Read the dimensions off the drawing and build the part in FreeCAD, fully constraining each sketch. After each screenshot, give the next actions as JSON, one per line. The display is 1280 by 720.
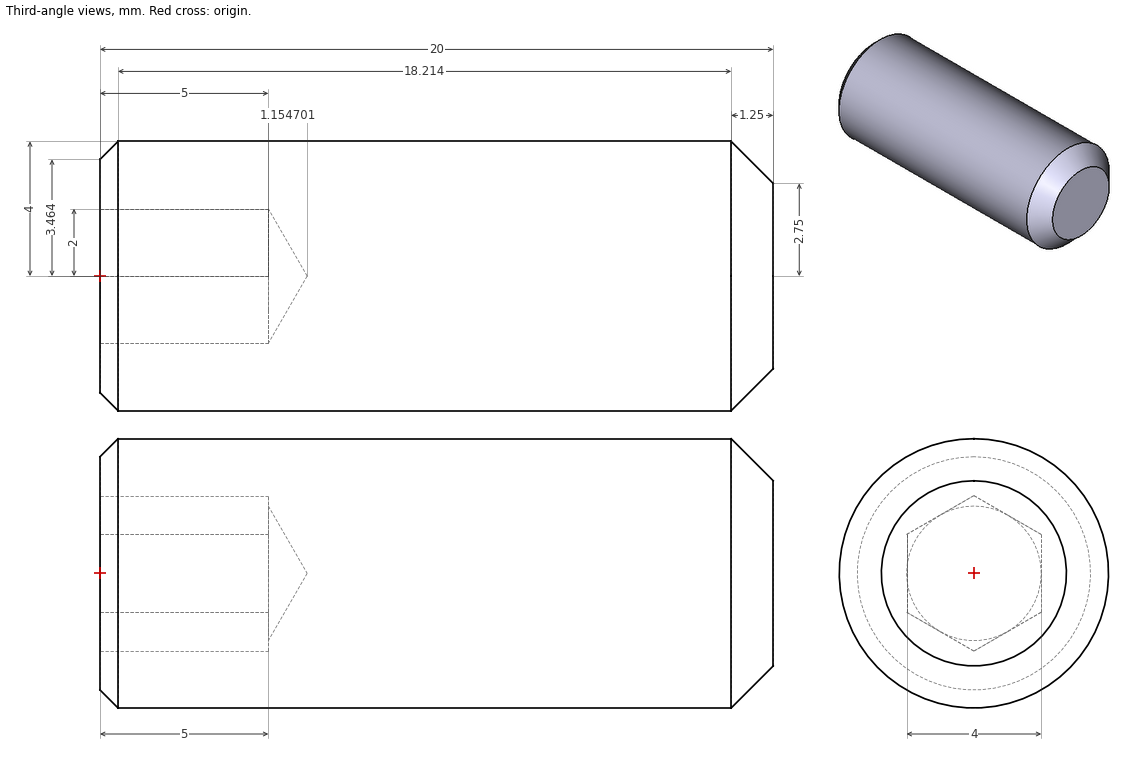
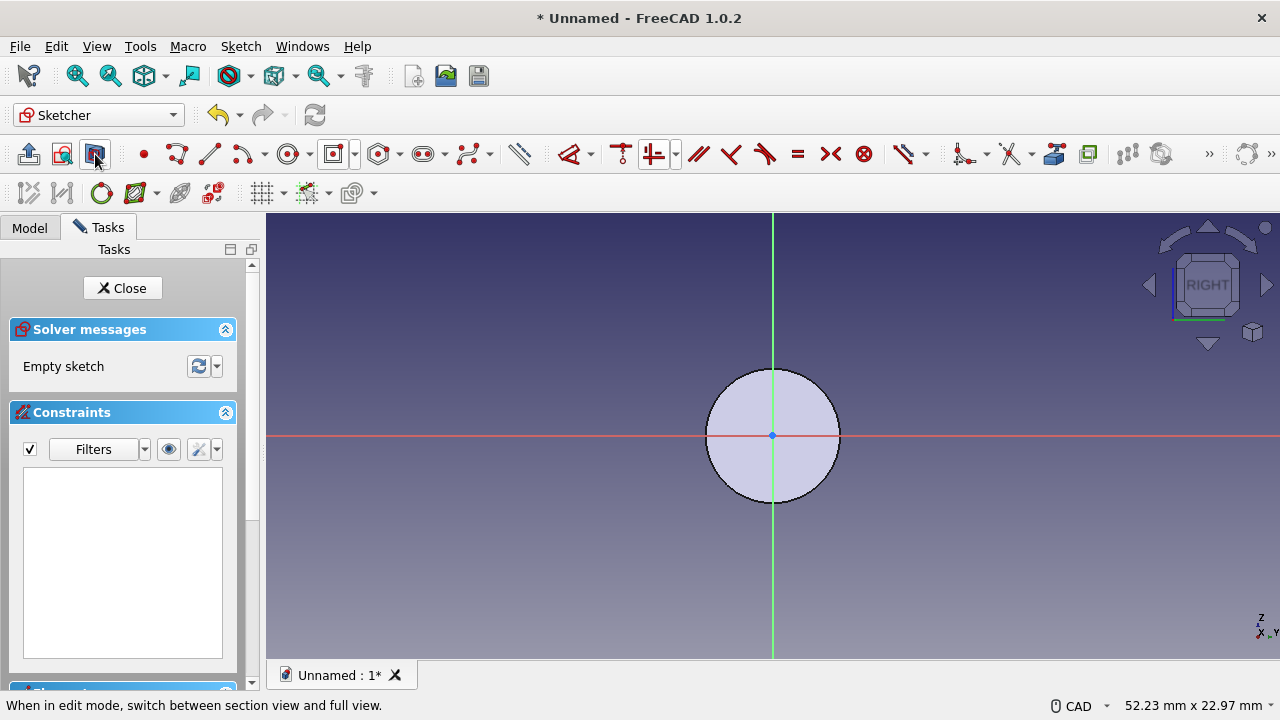
{"action": "scroll", "coordinate": [802, 436], "scroll_direction": "up", "scroll_amount": 6}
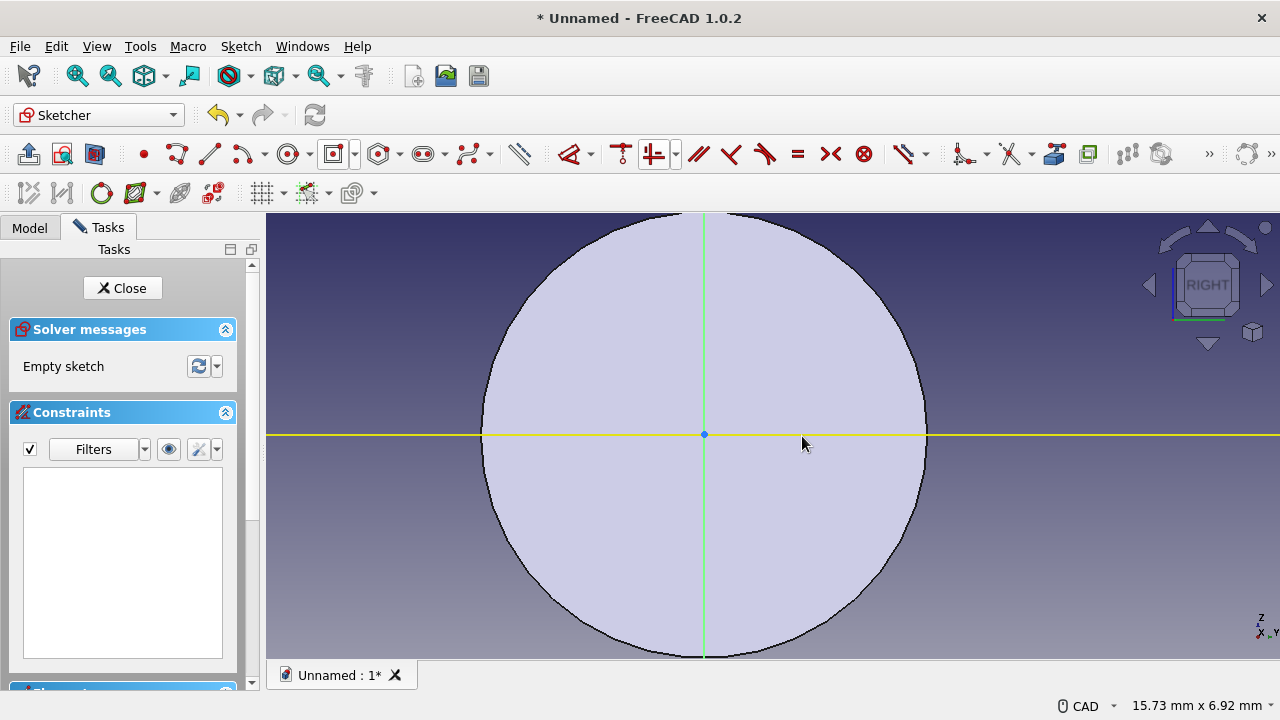
{"action": "left_click", "coordinate": [378, 154]}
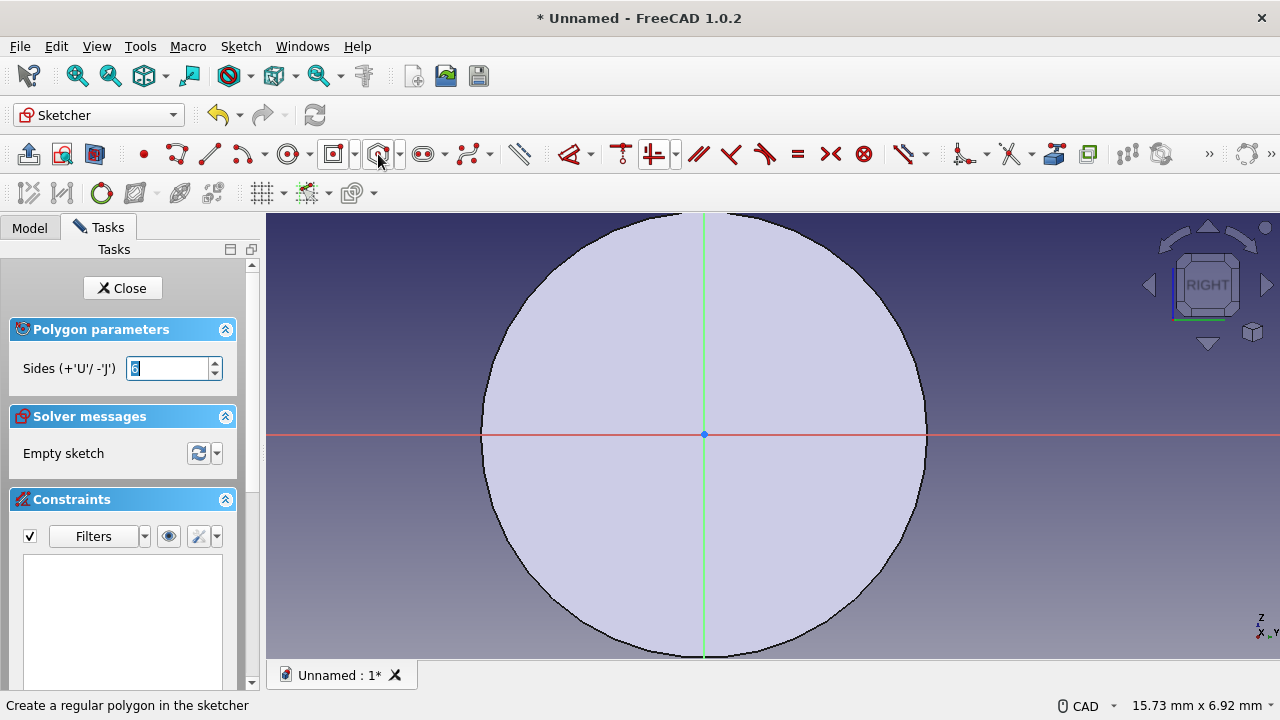
{"action": "left_click", "coordinate": [704, 435]}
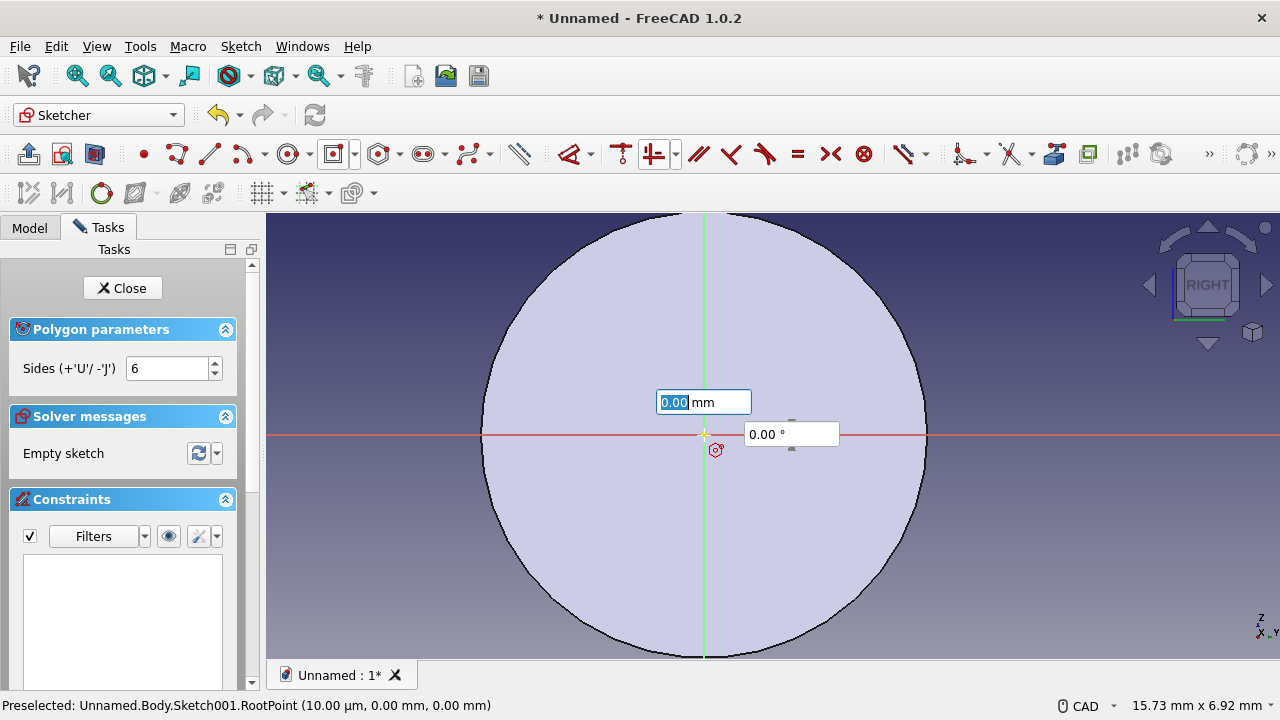
{"action": "left_click", "coordinate": [704, 286]}
{"action": "right_click", "coordinate": [704, 286]}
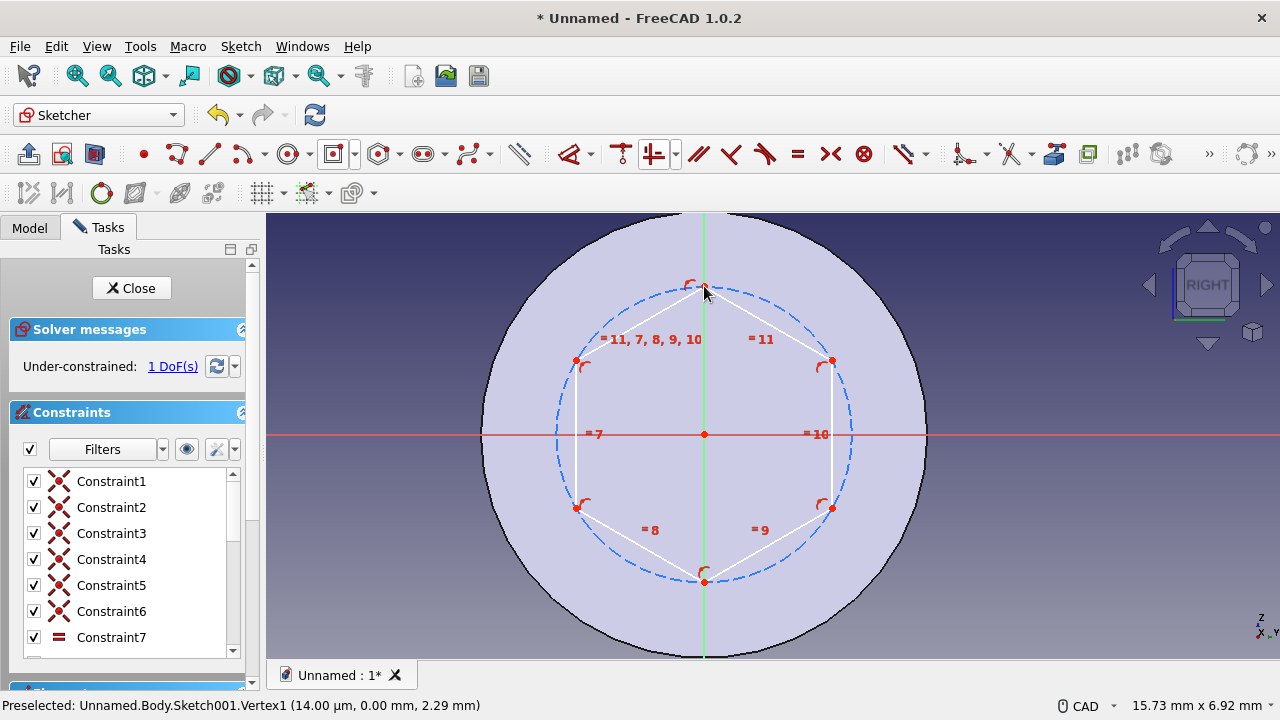
{"action": "left_click", "coordinate": [568, 154]}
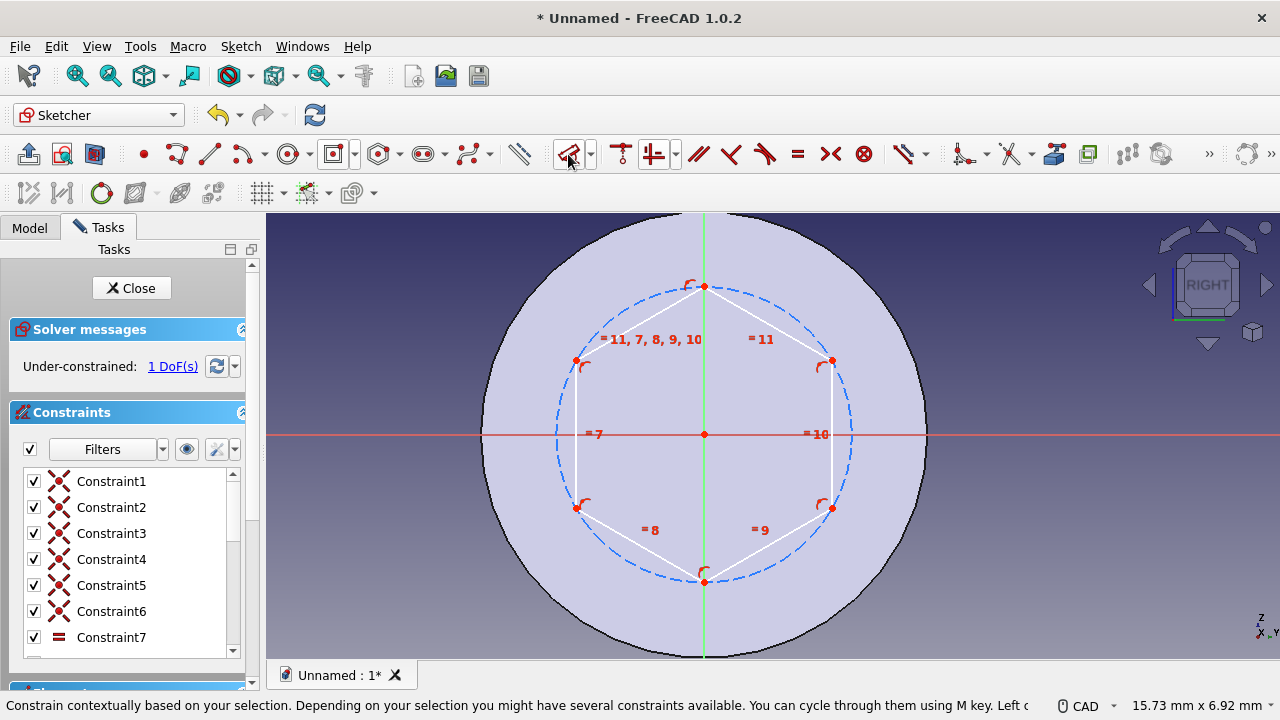
{"action": "left_click", "coordinate": [576, 361]}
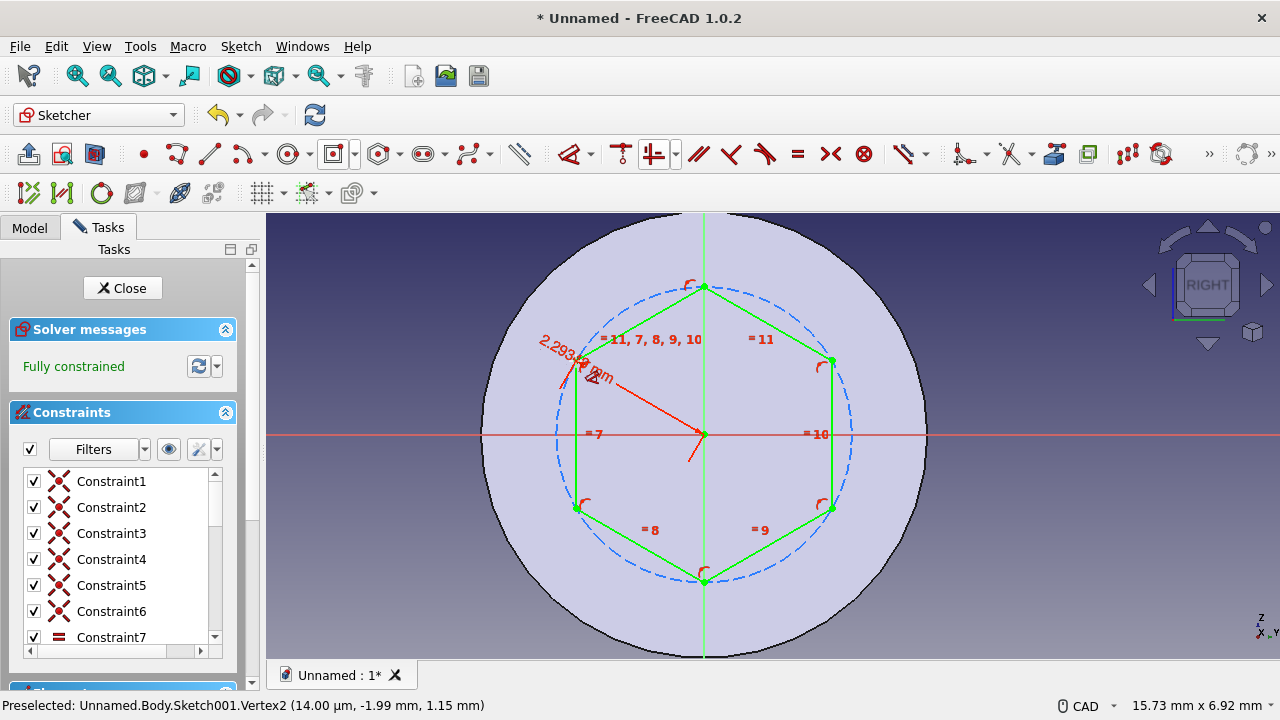
{"action": "left_click", "coordinate": [832, 509]}
{"action": "left_click", "coordinate": [645, 591]}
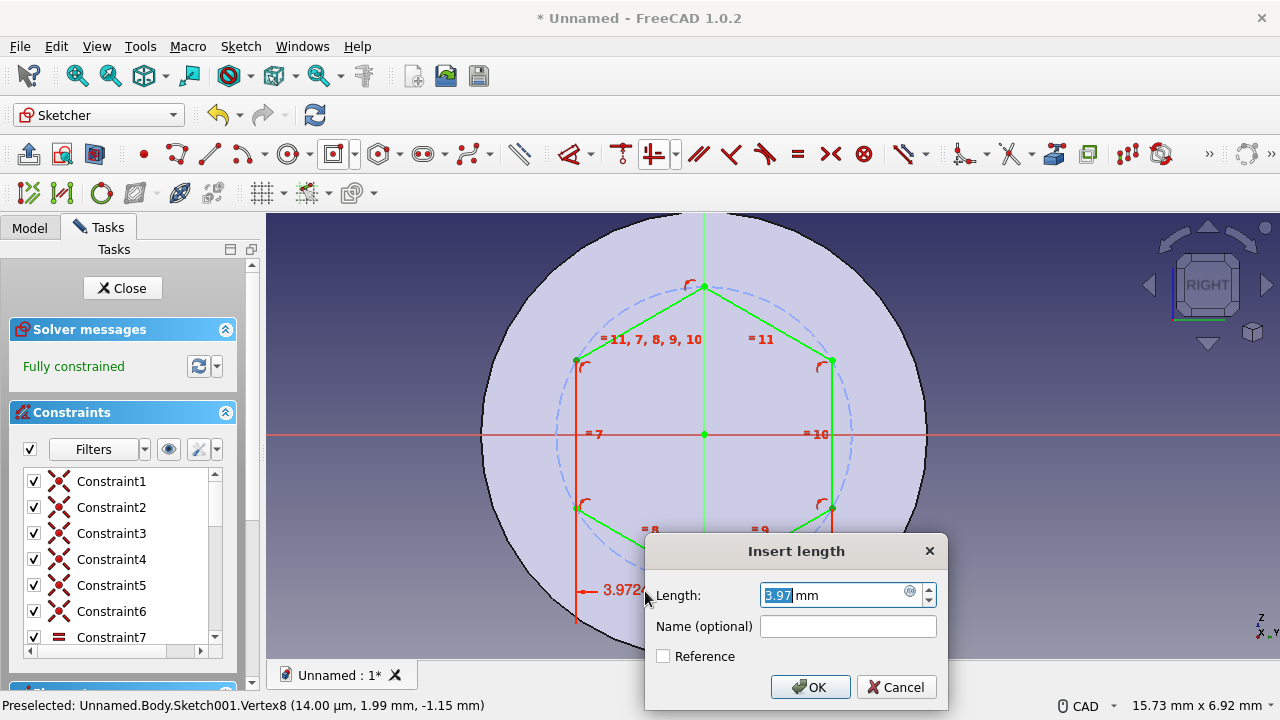
{"action": "type", "text": "4"}
{"action": "key", "text": "Return"}
{"action": "key", "text": "Escape"}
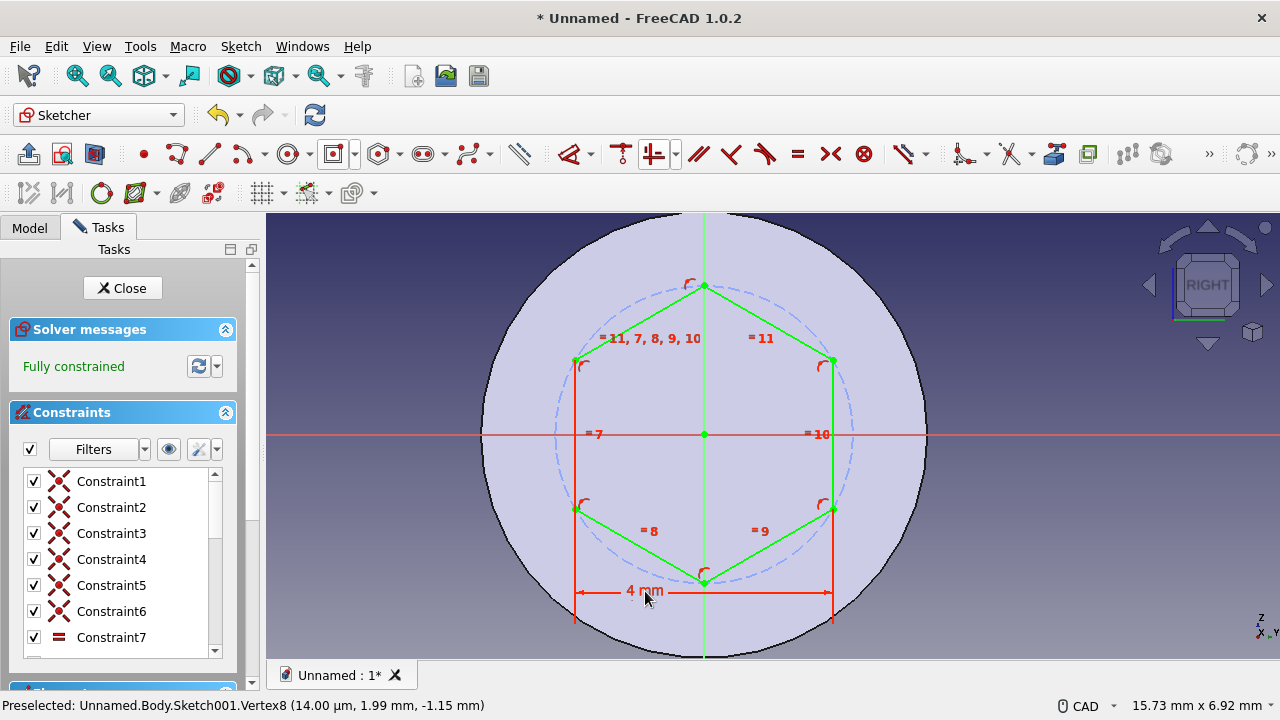
{"action": "left_click", "coordinate": [123, 288]}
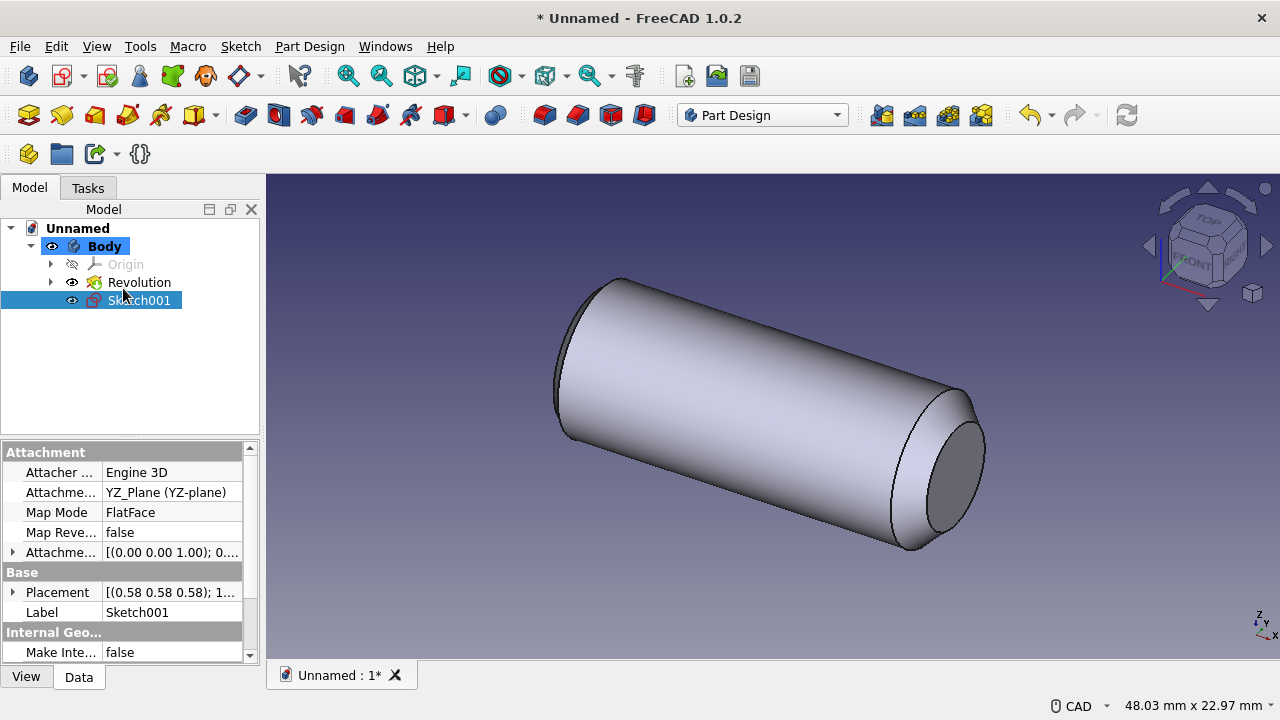
{"action": "left_click", "coordinate": [246, 116]}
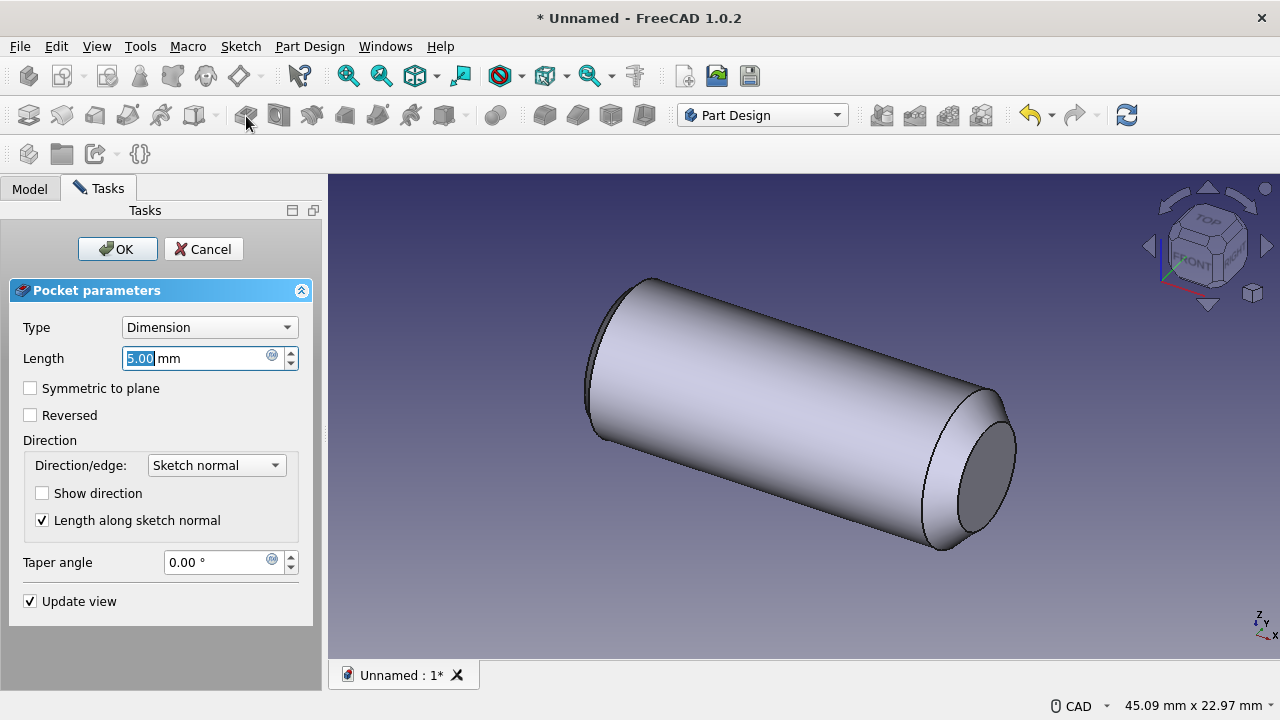
{"action": "type", "text": "5"}
{"action": "key", "text": "Tab"}